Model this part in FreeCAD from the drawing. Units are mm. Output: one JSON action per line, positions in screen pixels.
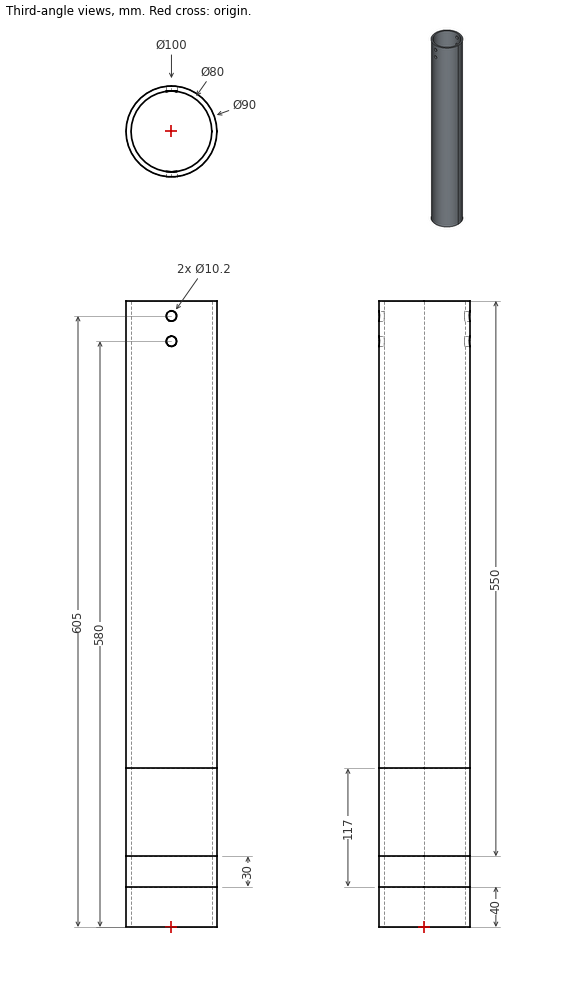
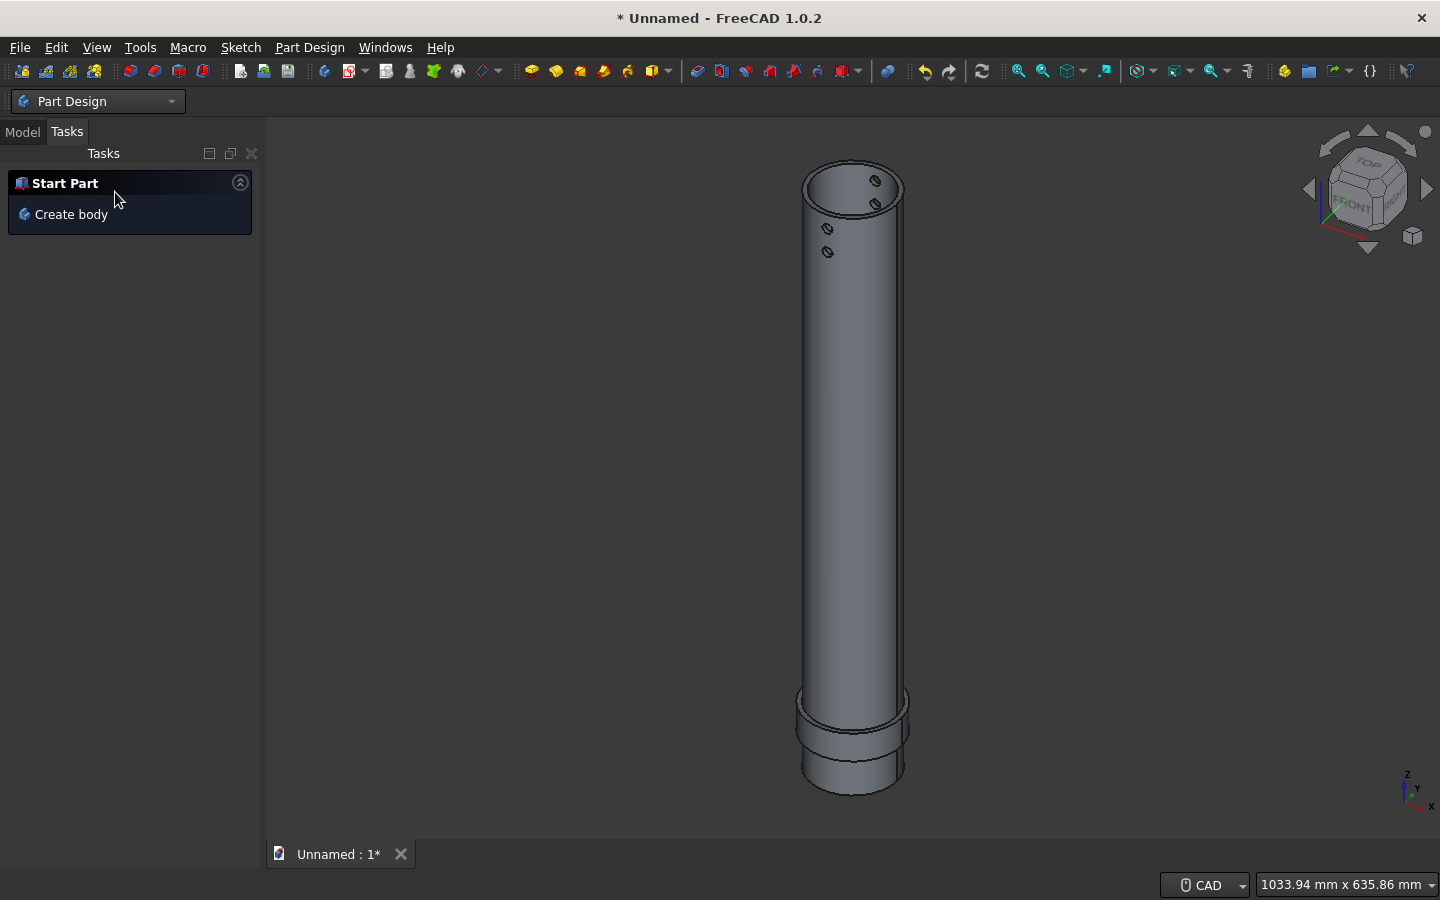
{"action": "key", "text": "5"}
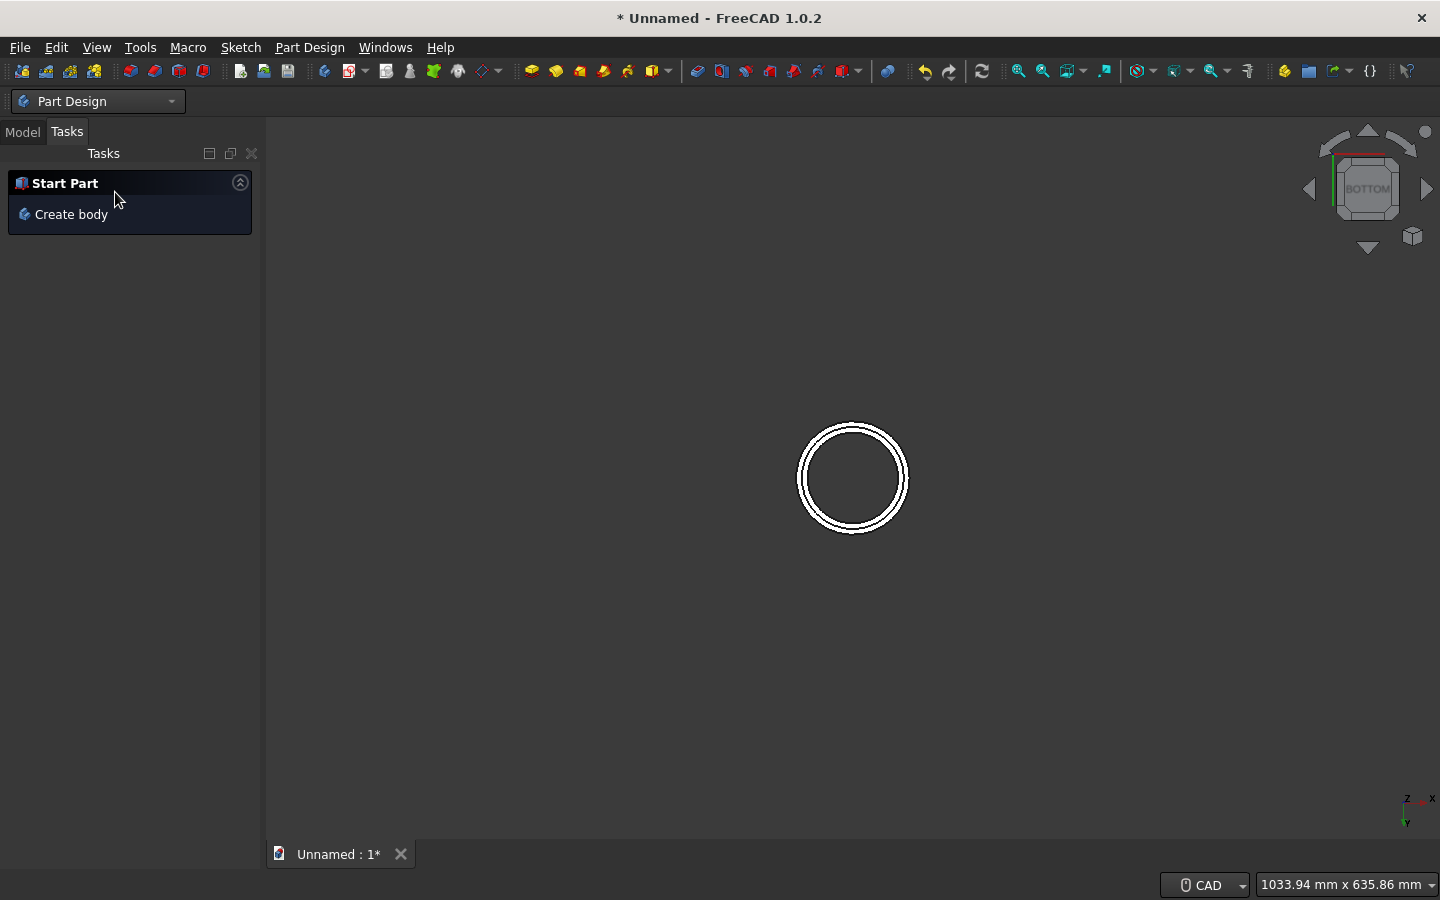
{"action": "left_click", "coordinate": [1020, 72]}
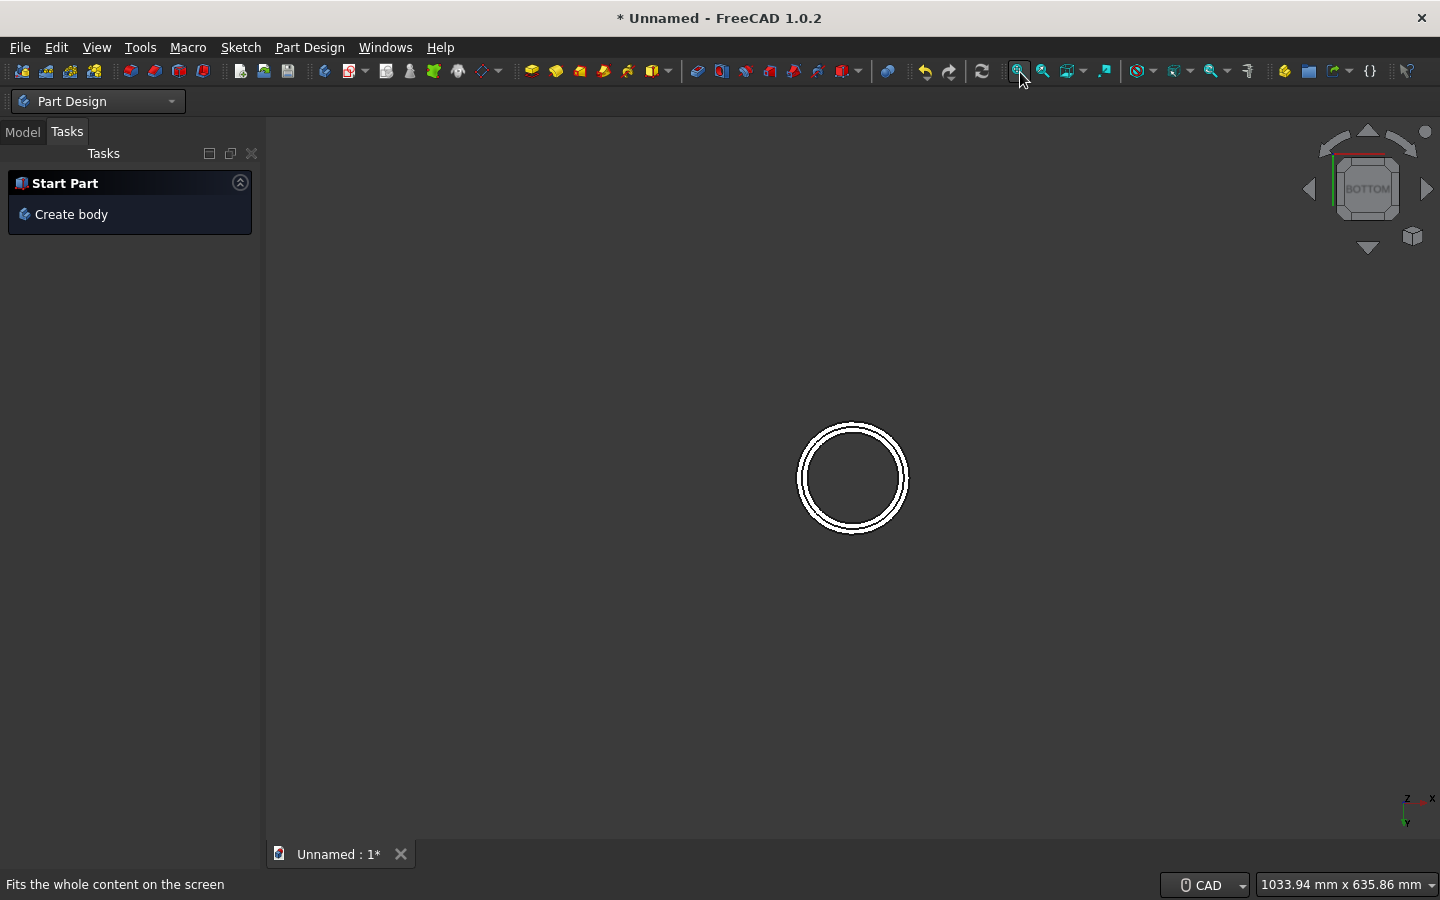
{"action": "scroll", "coordinate": [869, 526], "scroll_direction": "up", "scroll_amount": 15}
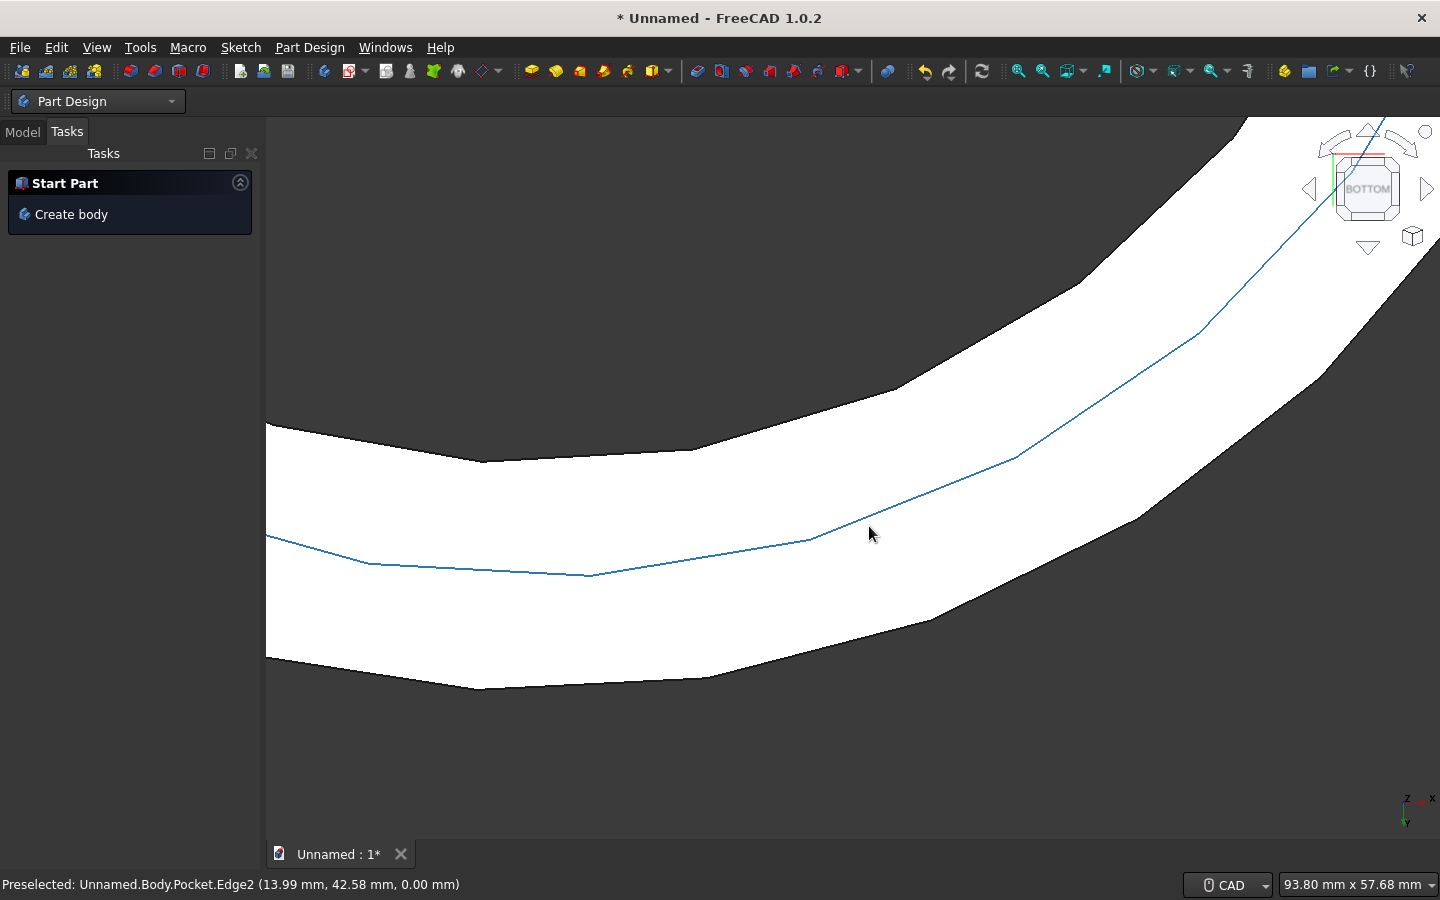
{"action": "scroll", "coordinate": [861, 527], "scroll_direction": "up", "scroll_amount": 6}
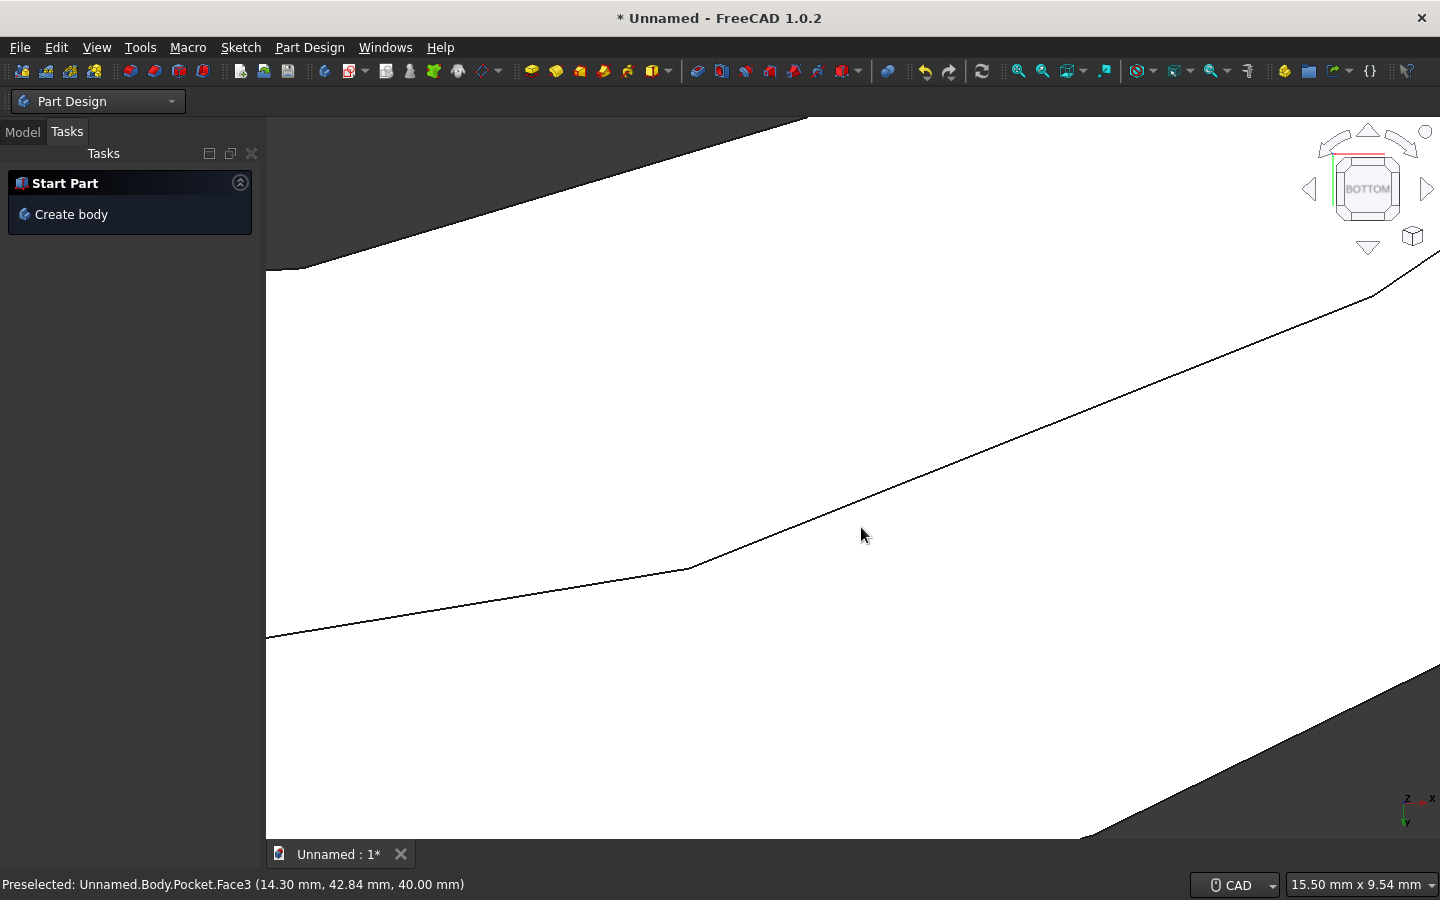
{"action": "left_click", "coordinate": [859, 530]}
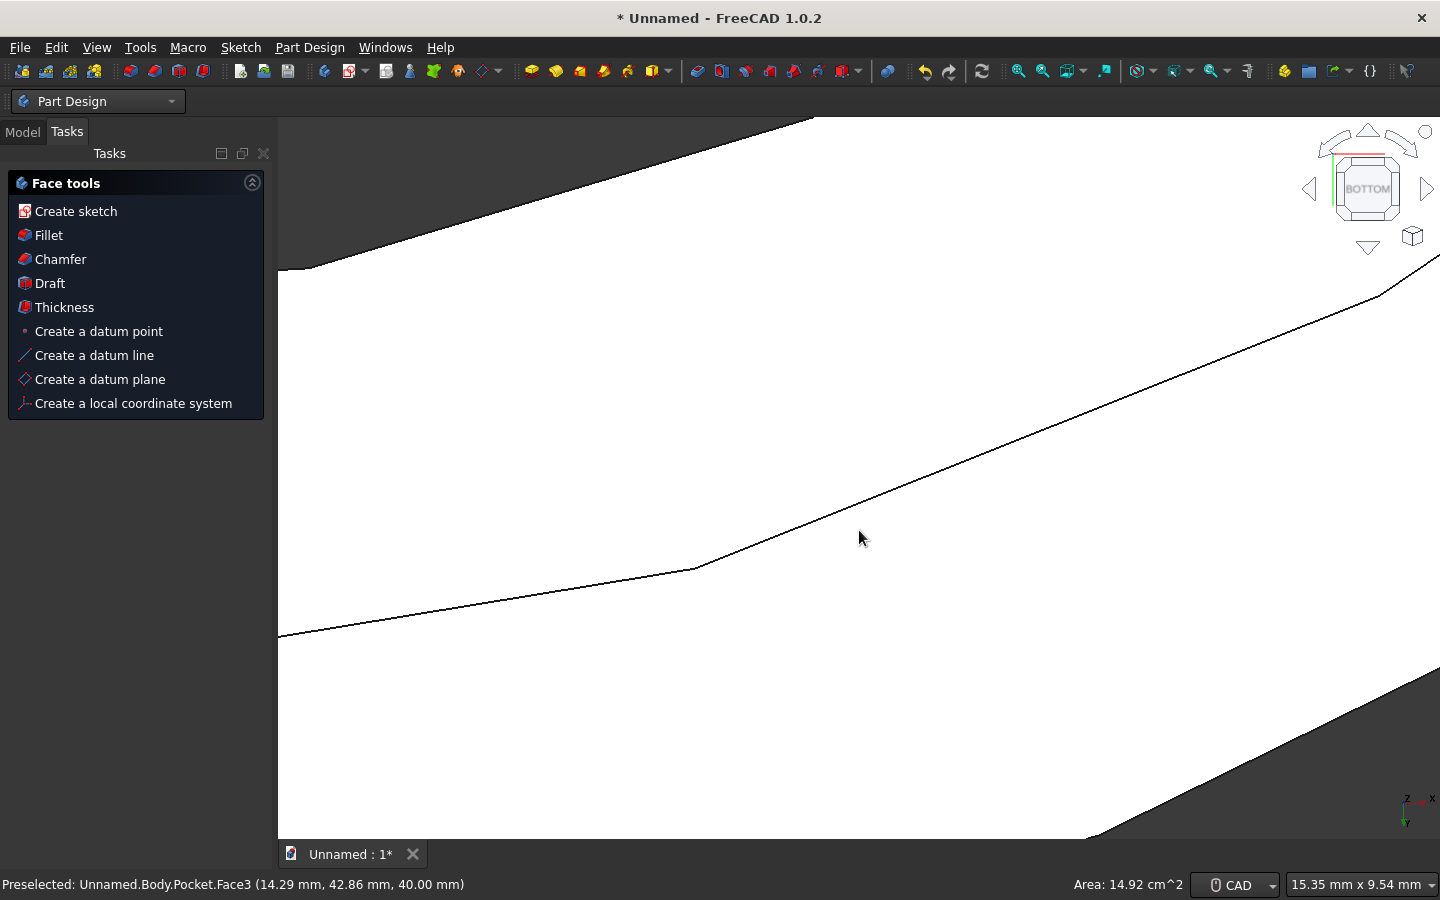
{"action": "left_click", "coordinate": [350, 72]}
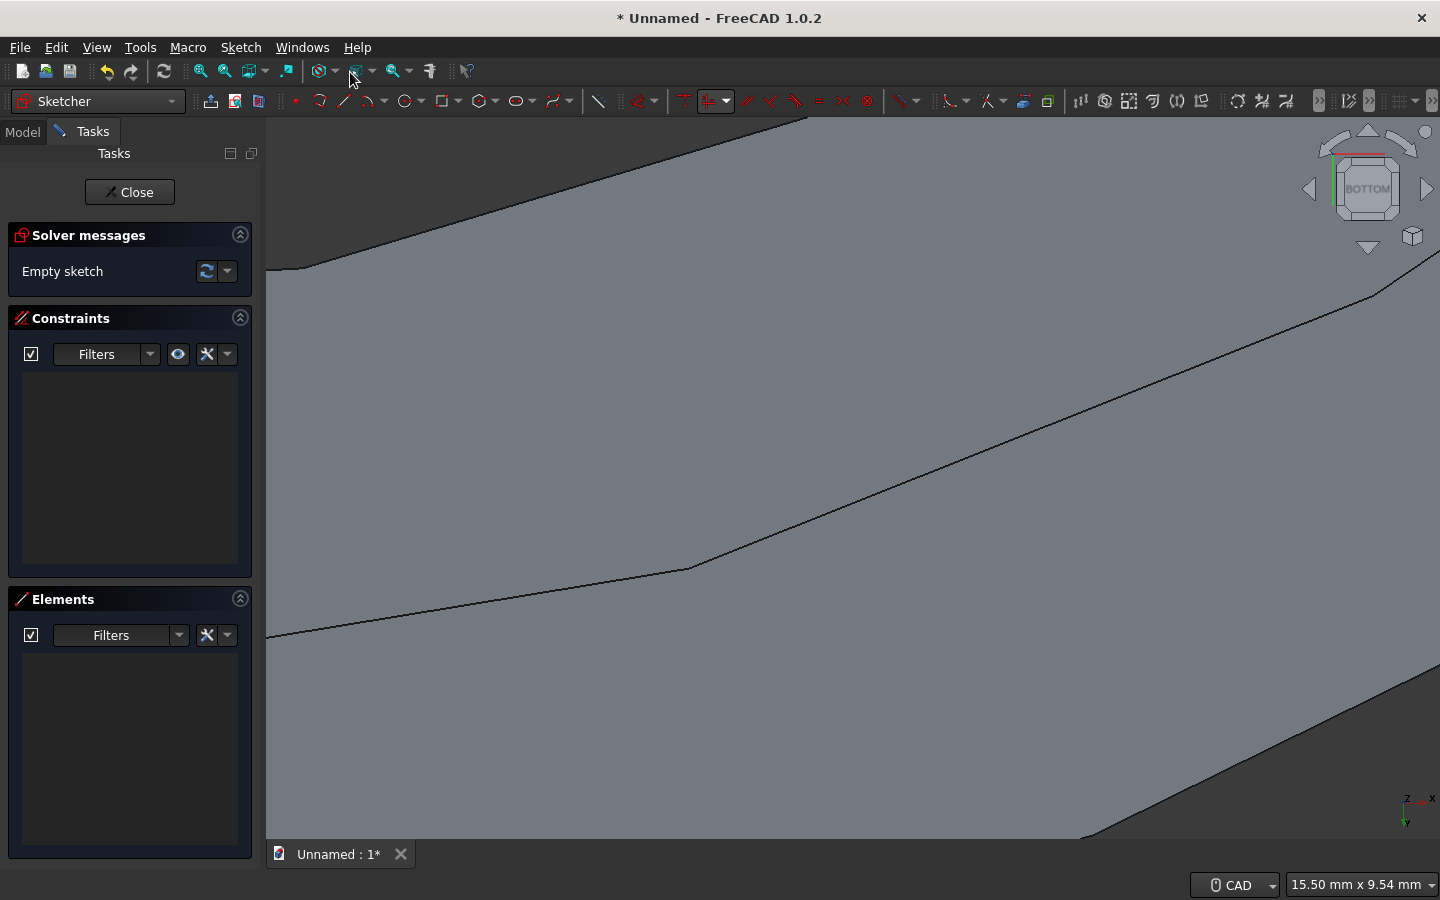
{"action": "scroll", "coordinate": [850, 685], "scroll_direction": "down", "scroll_amount": 14}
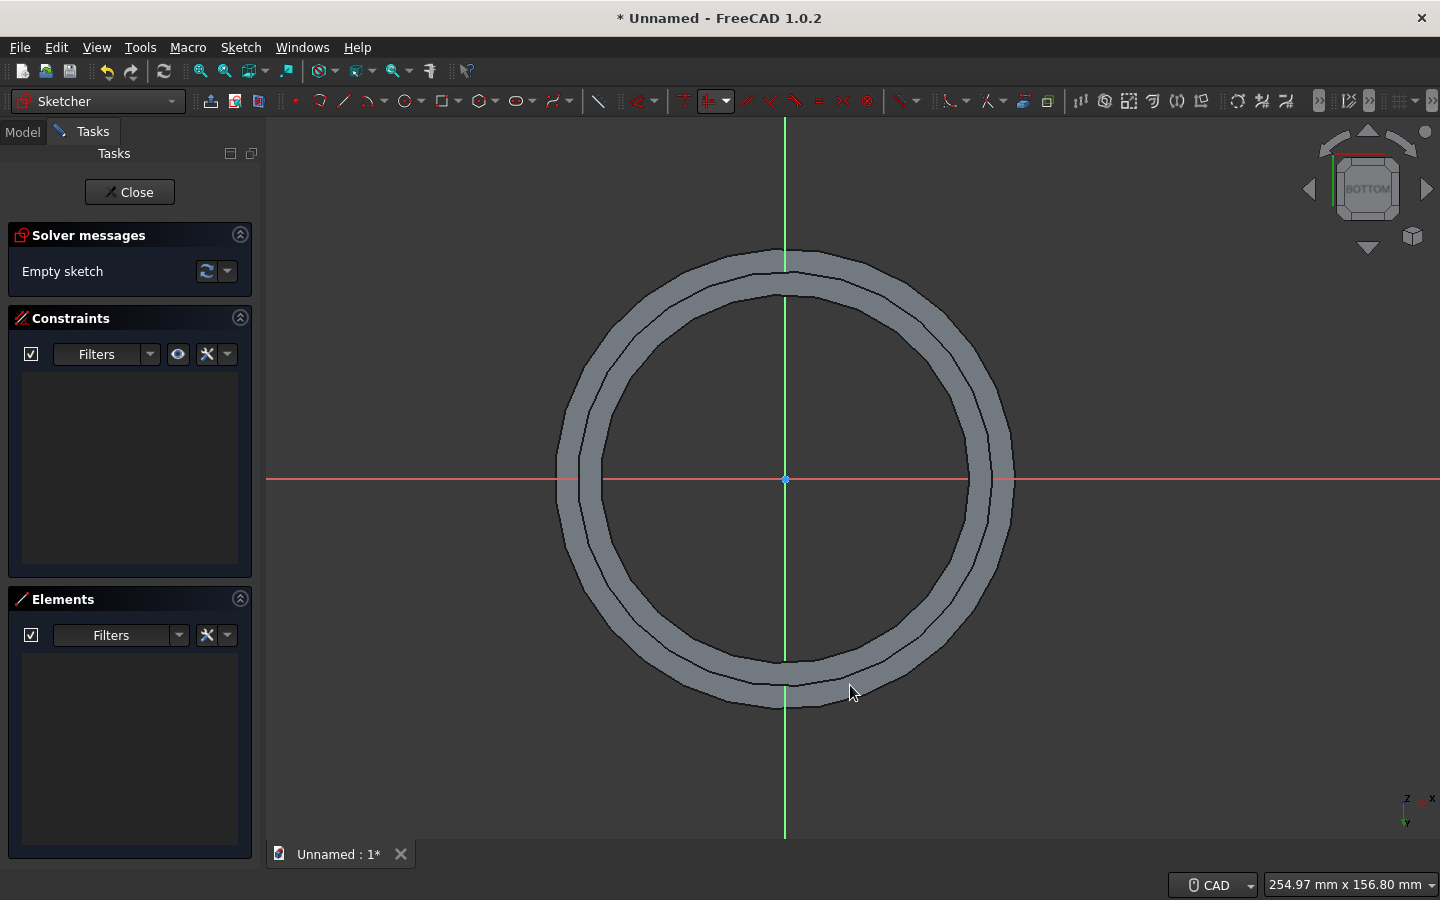
{"action": "key", "text": "g c"}